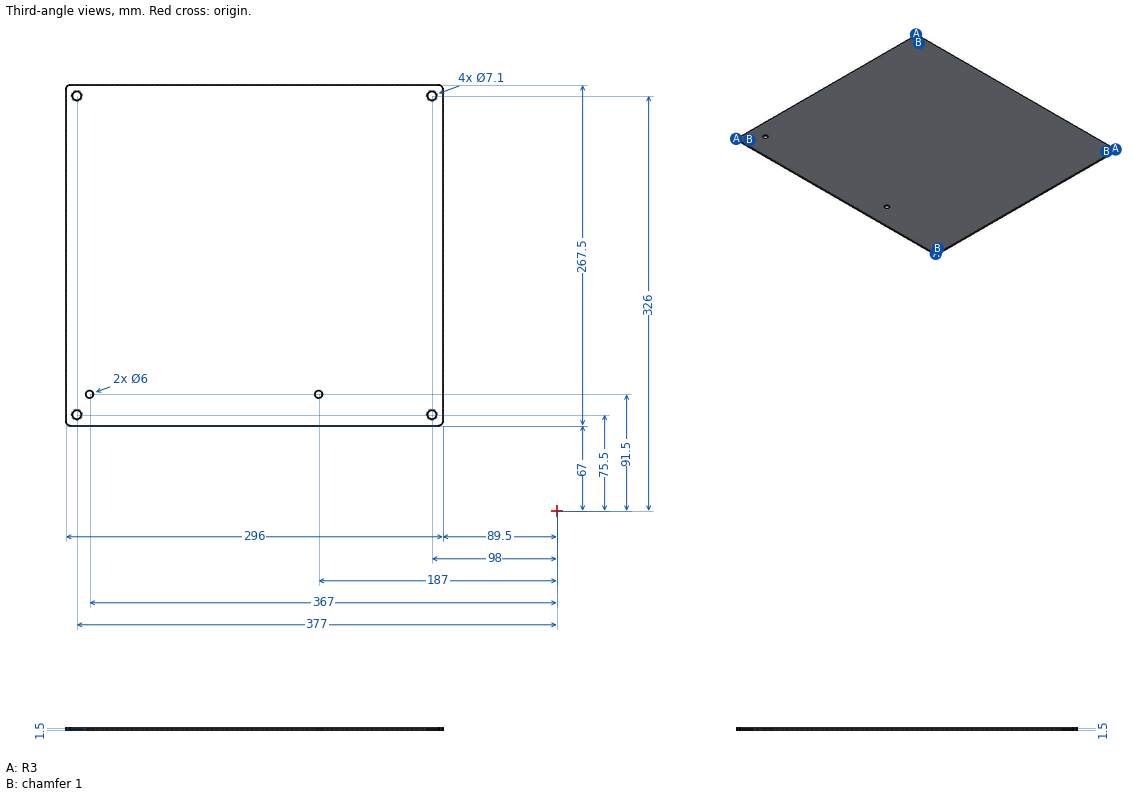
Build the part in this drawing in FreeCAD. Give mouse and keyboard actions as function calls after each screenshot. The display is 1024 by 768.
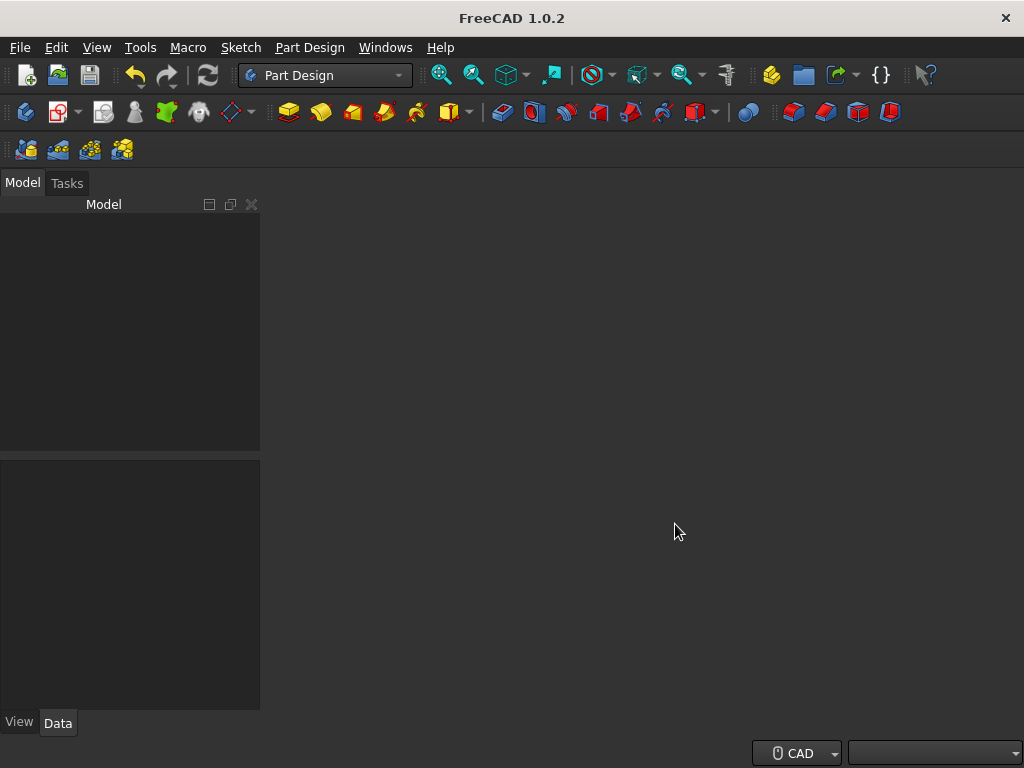
click(26, 76)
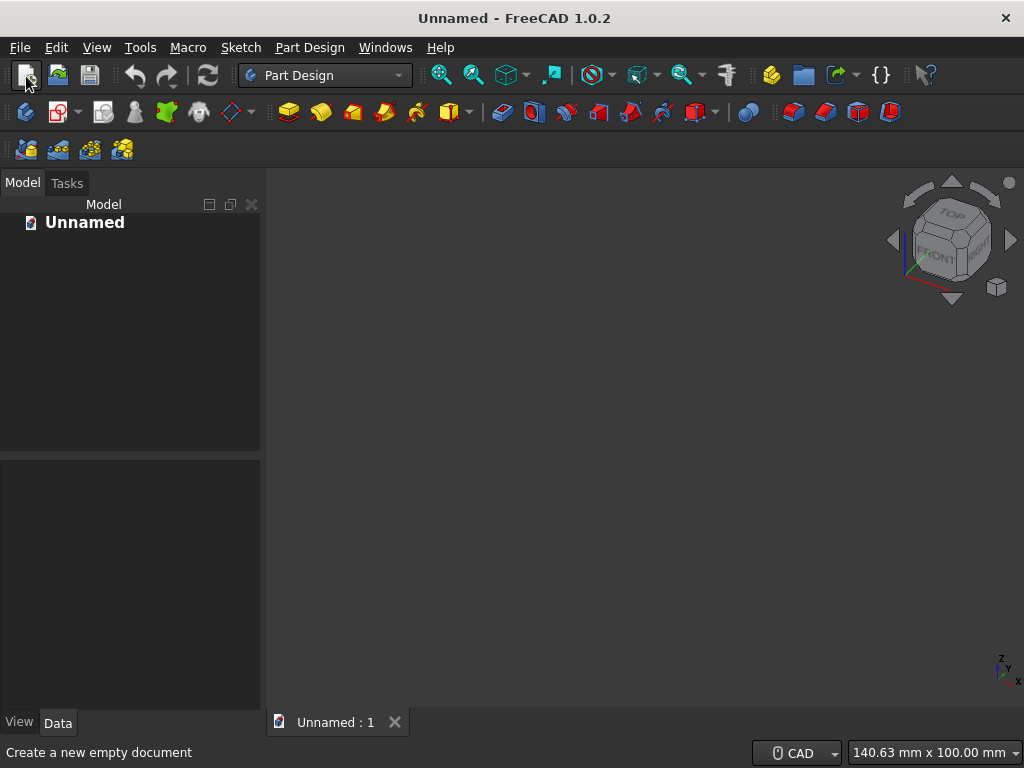
click(58, 112)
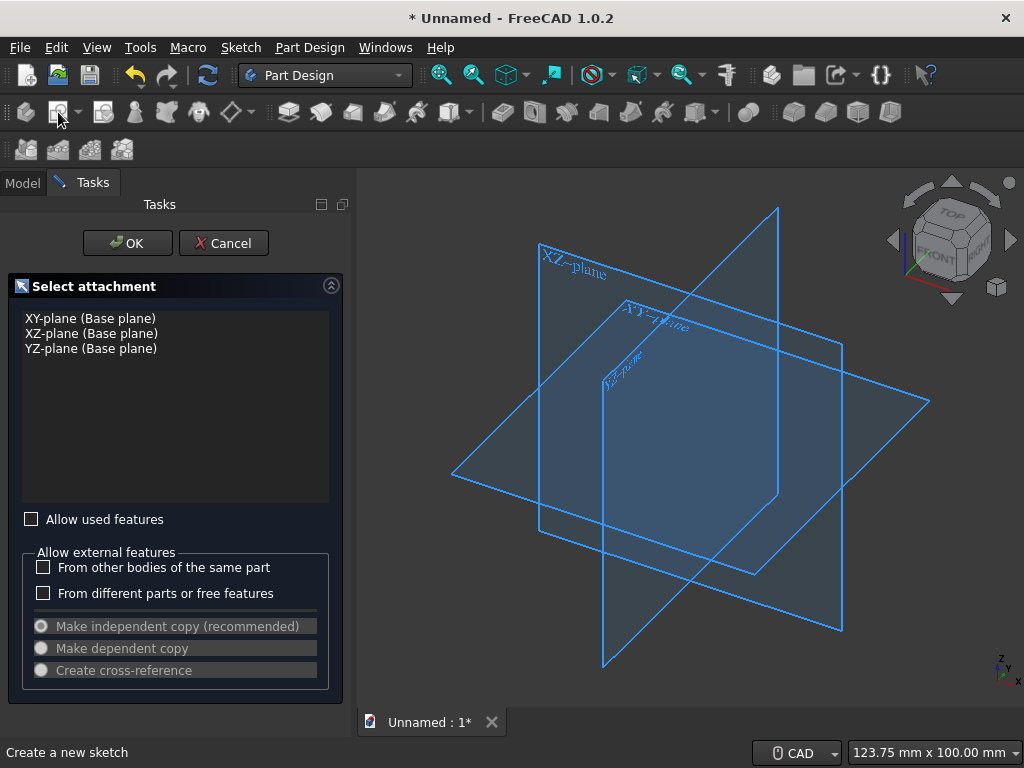
click(82, 318)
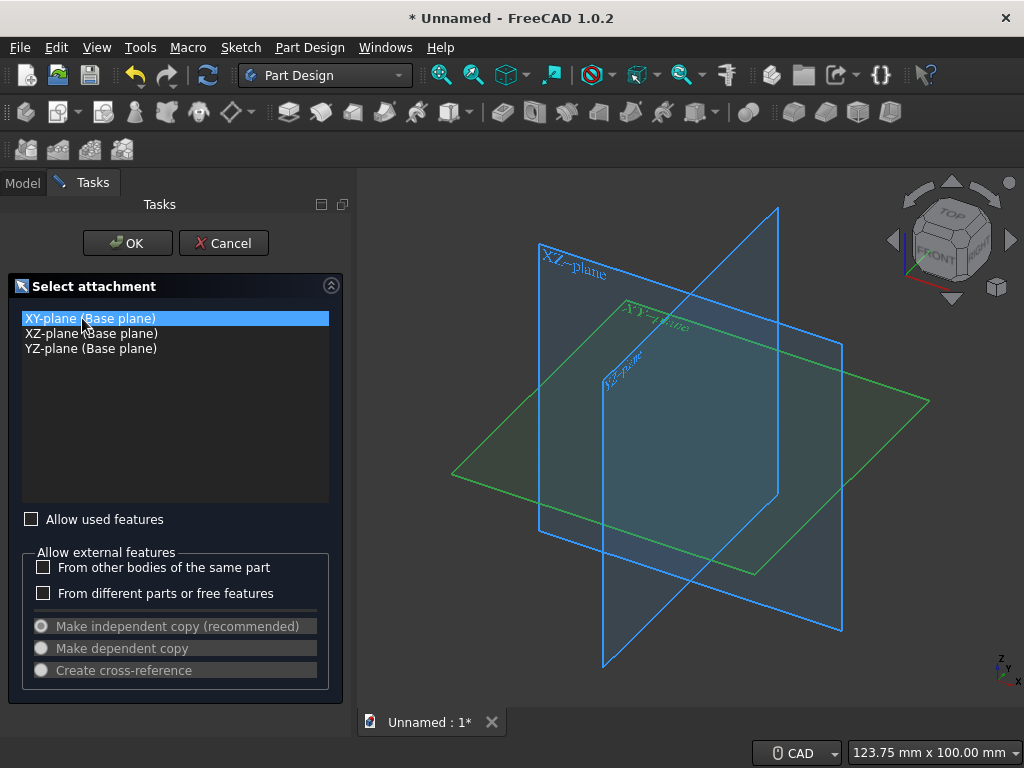
click(128, 243)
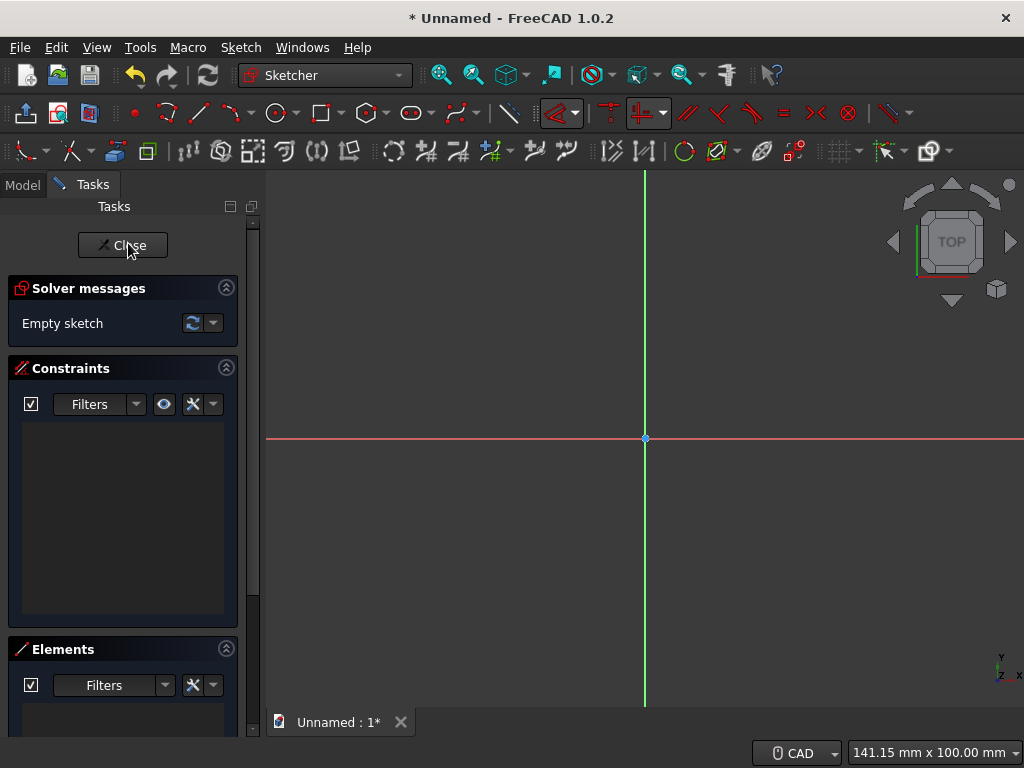
scroll(821, 666, down, 8)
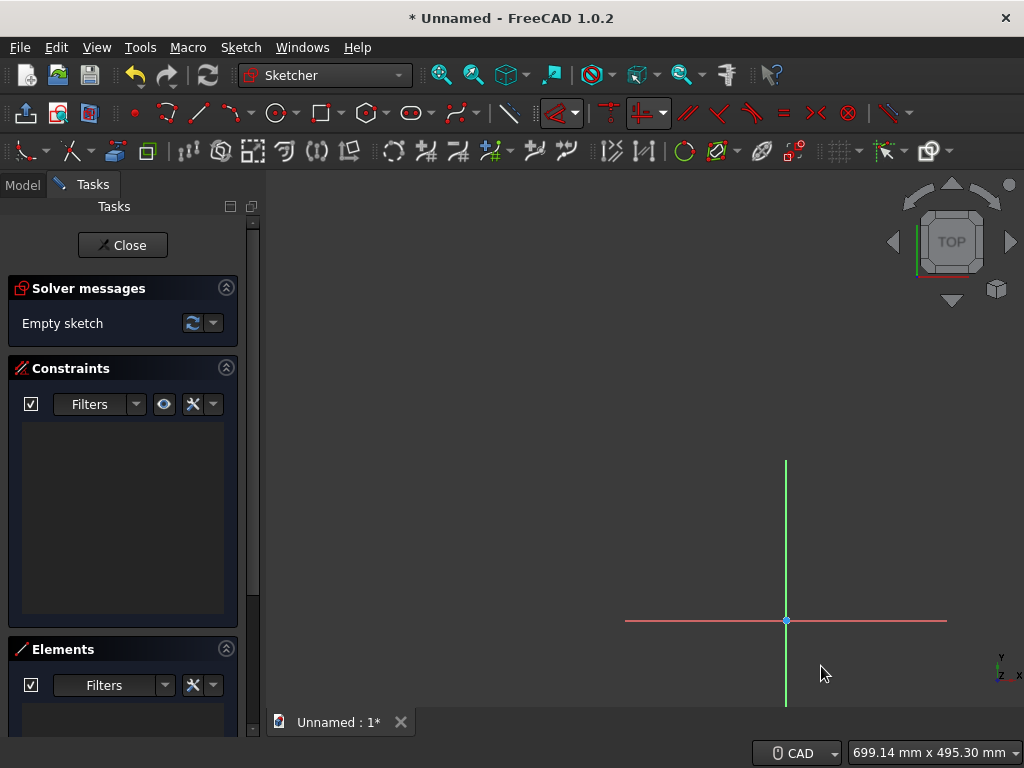
click(322, 114)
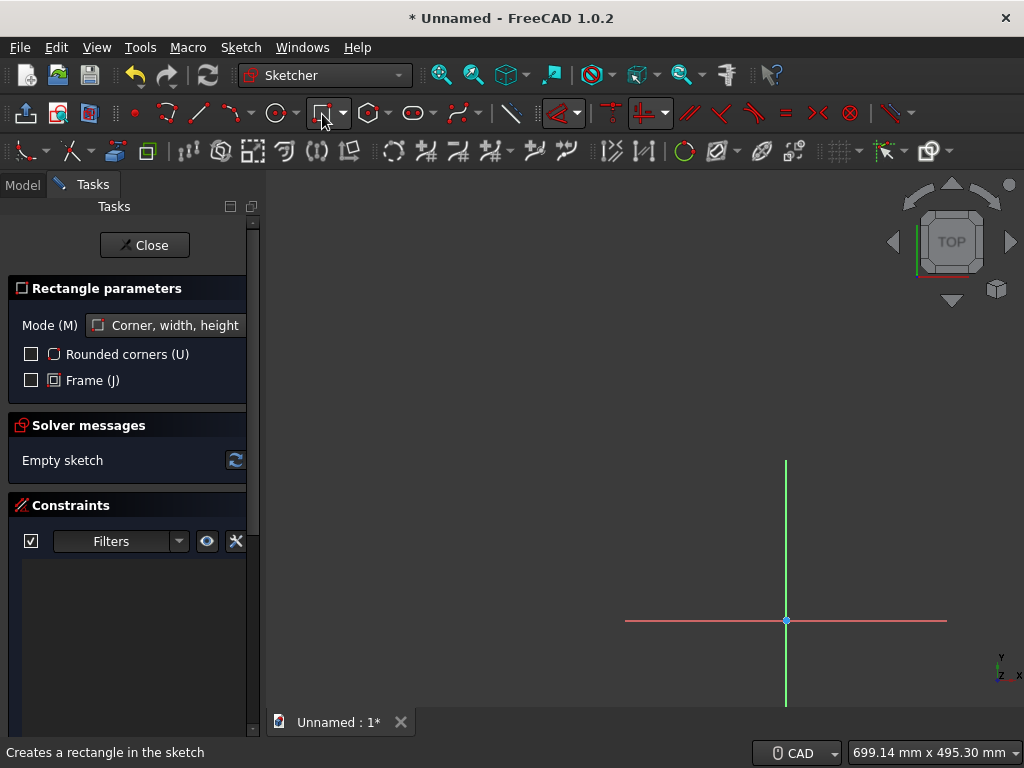
click(368, 258)
move(689, 548)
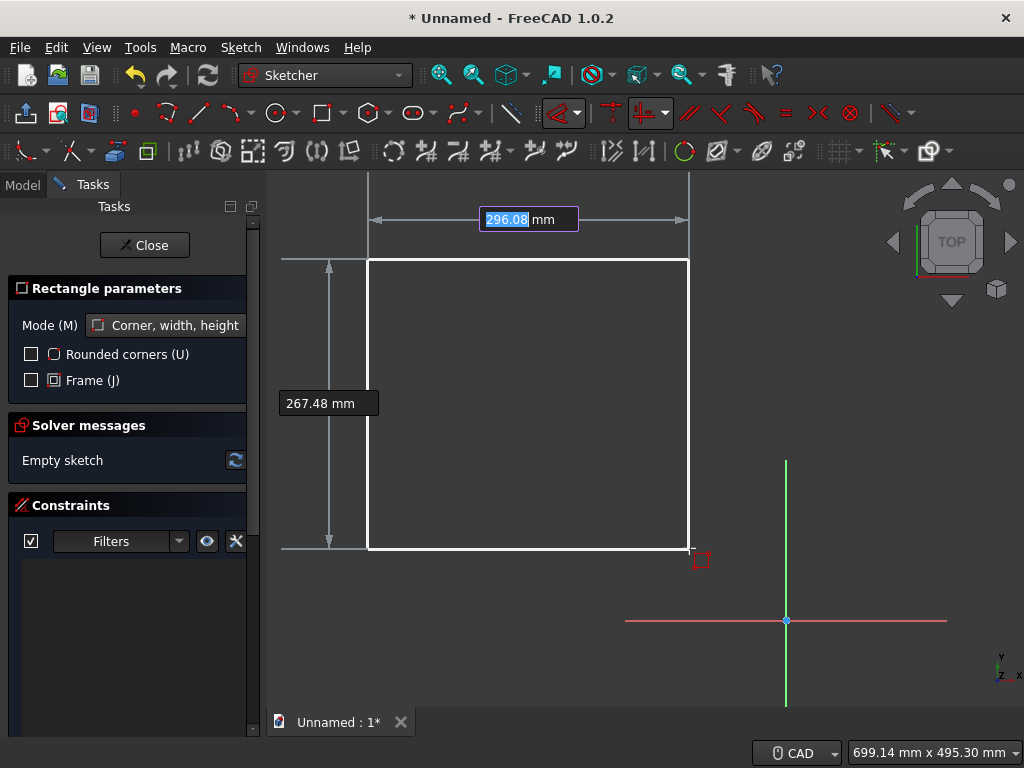
text(296)
key(Tab)
text(267.5)
key(Return)
key(Escape)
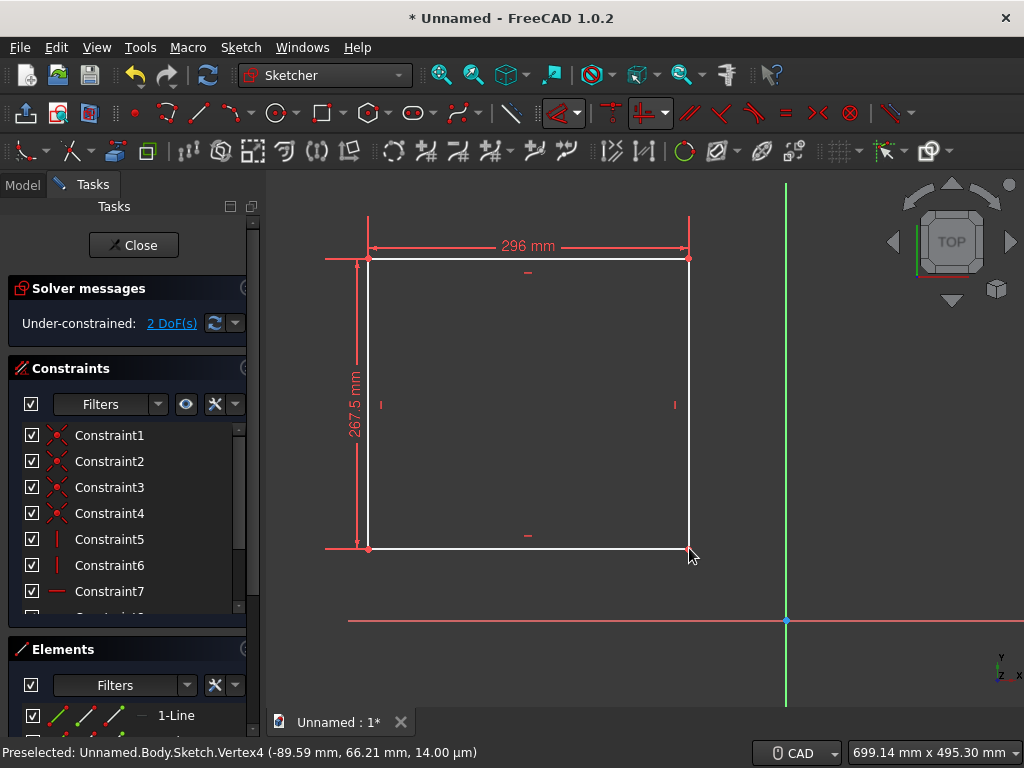
click(558, 114)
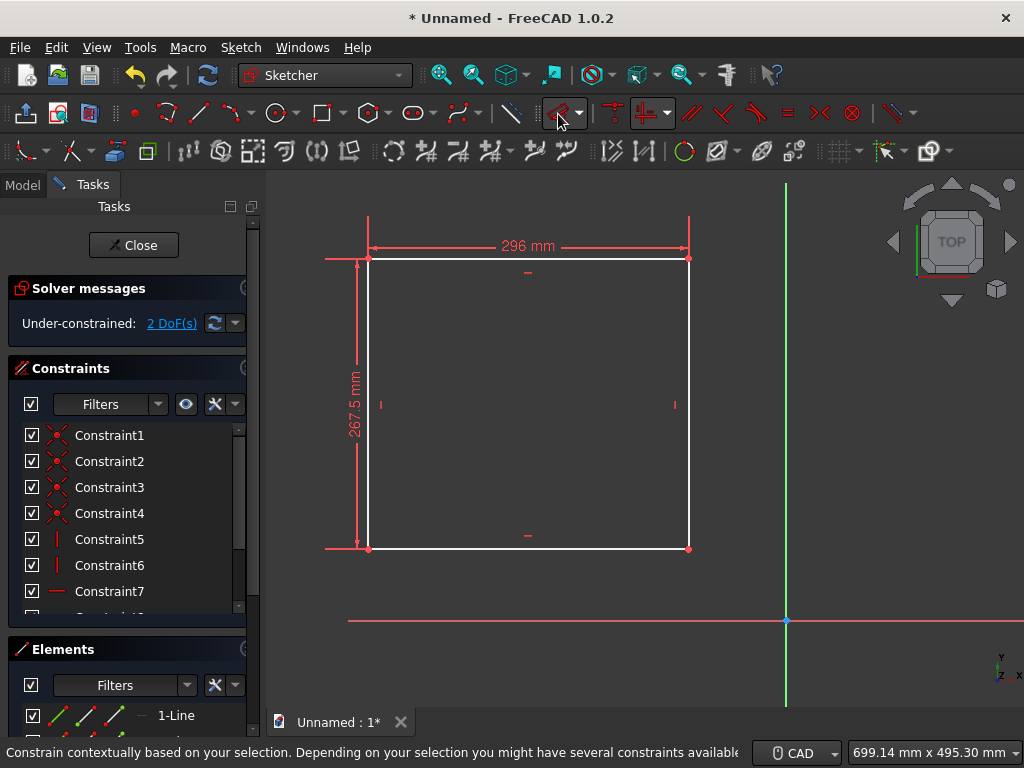
click(368, 549)
click(334, 585)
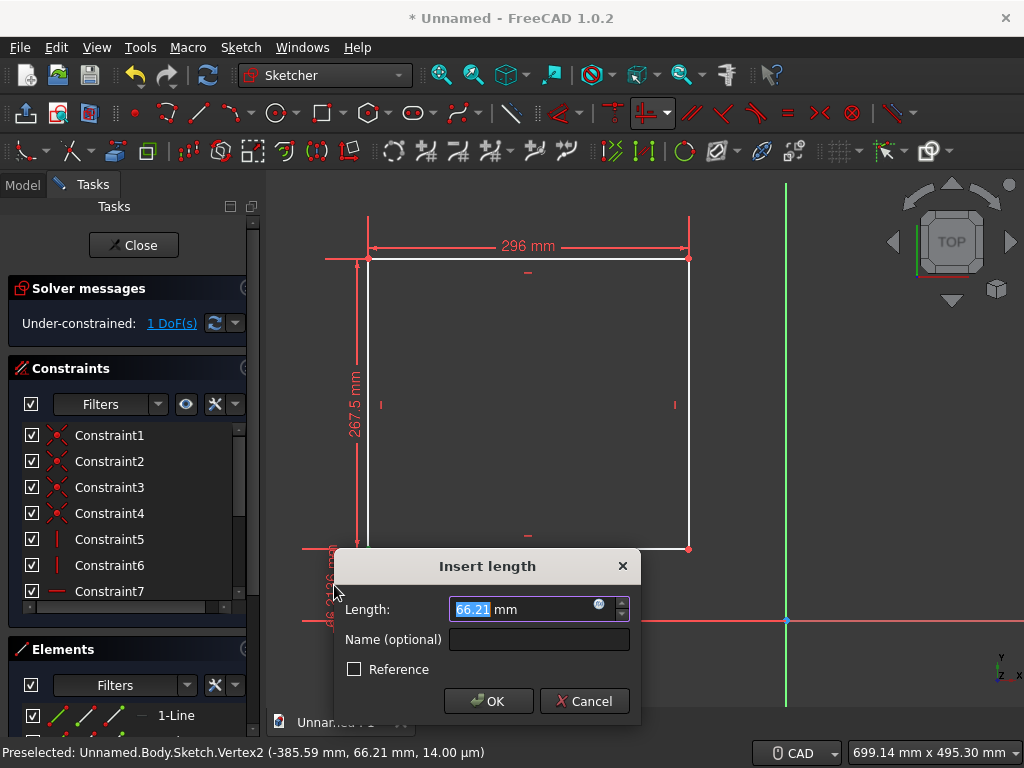
text(67)
key(Return)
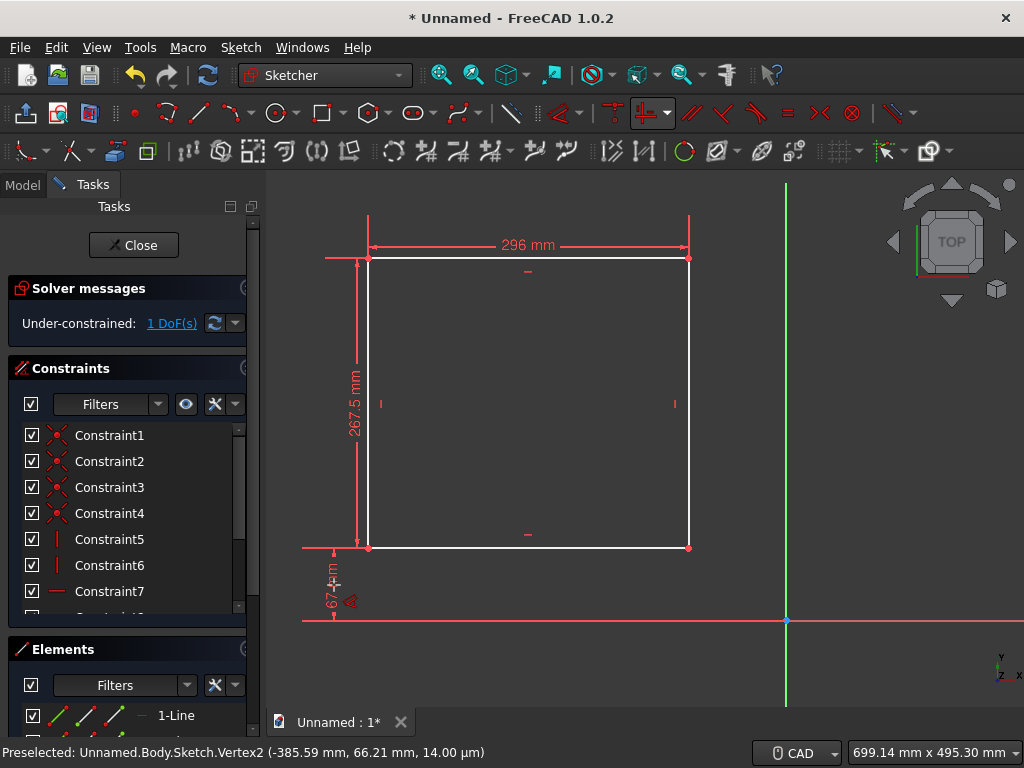
click(689, 548)
click(737, 655)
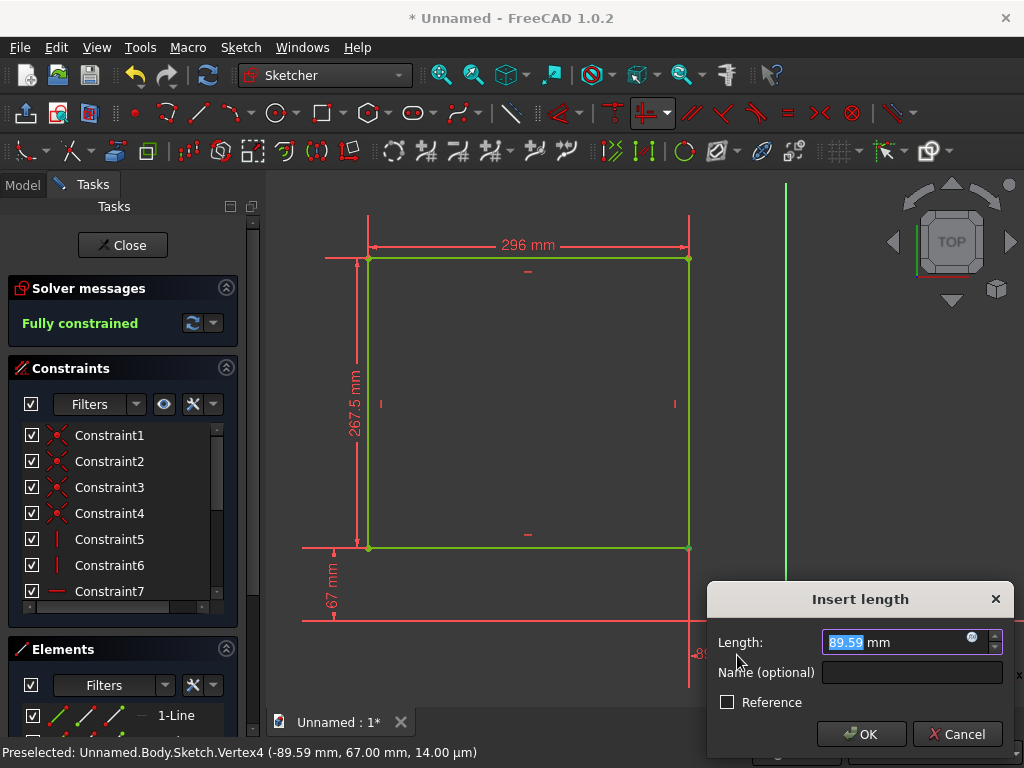
text(89.5)
key(Return)
key(Escape)